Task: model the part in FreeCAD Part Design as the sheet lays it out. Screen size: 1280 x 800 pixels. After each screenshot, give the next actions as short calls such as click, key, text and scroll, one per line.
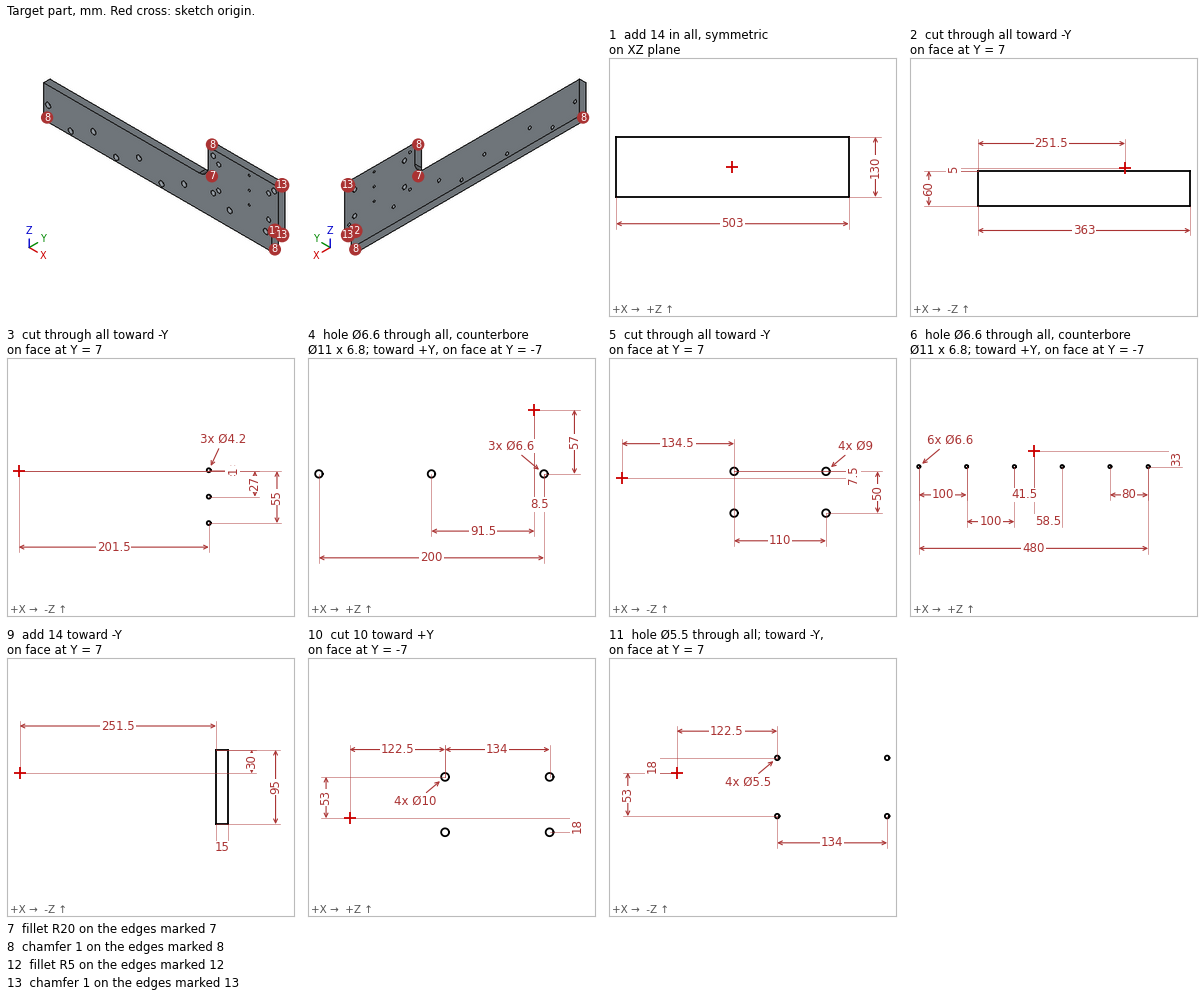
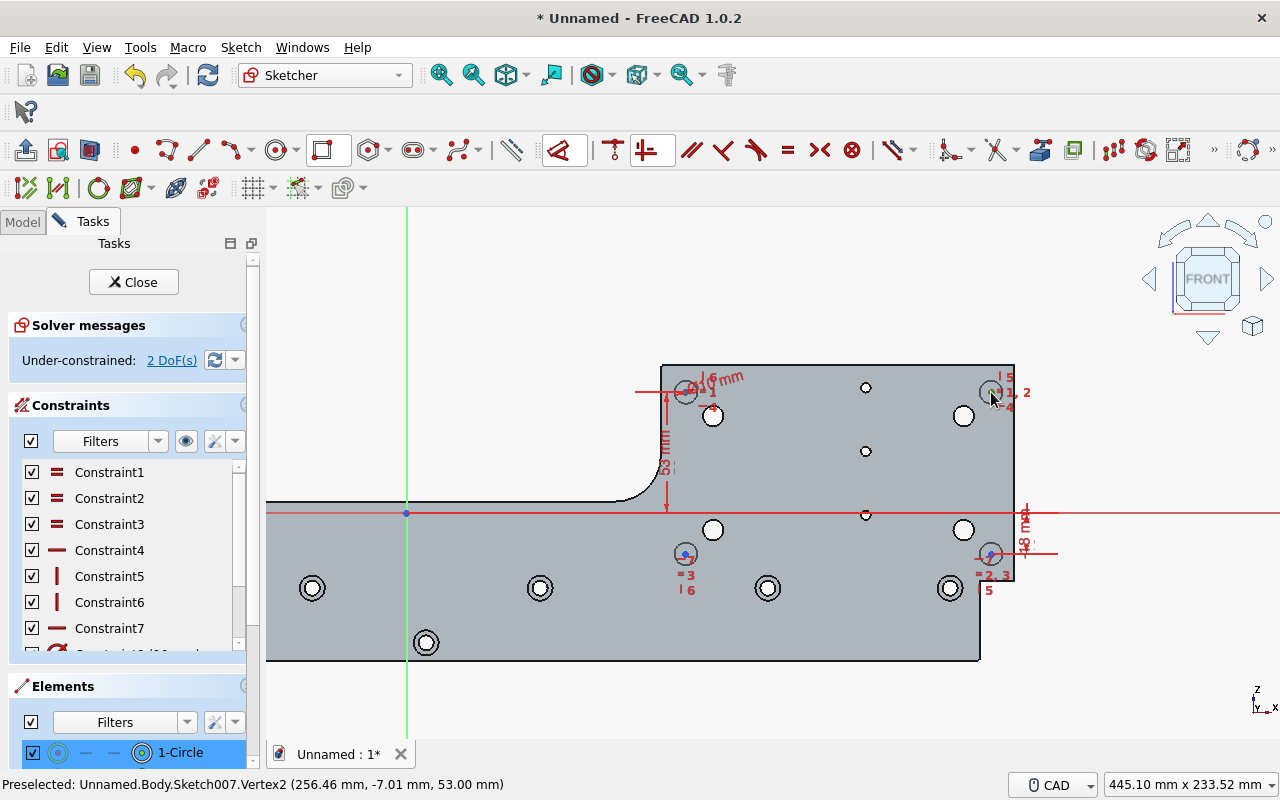
key(l)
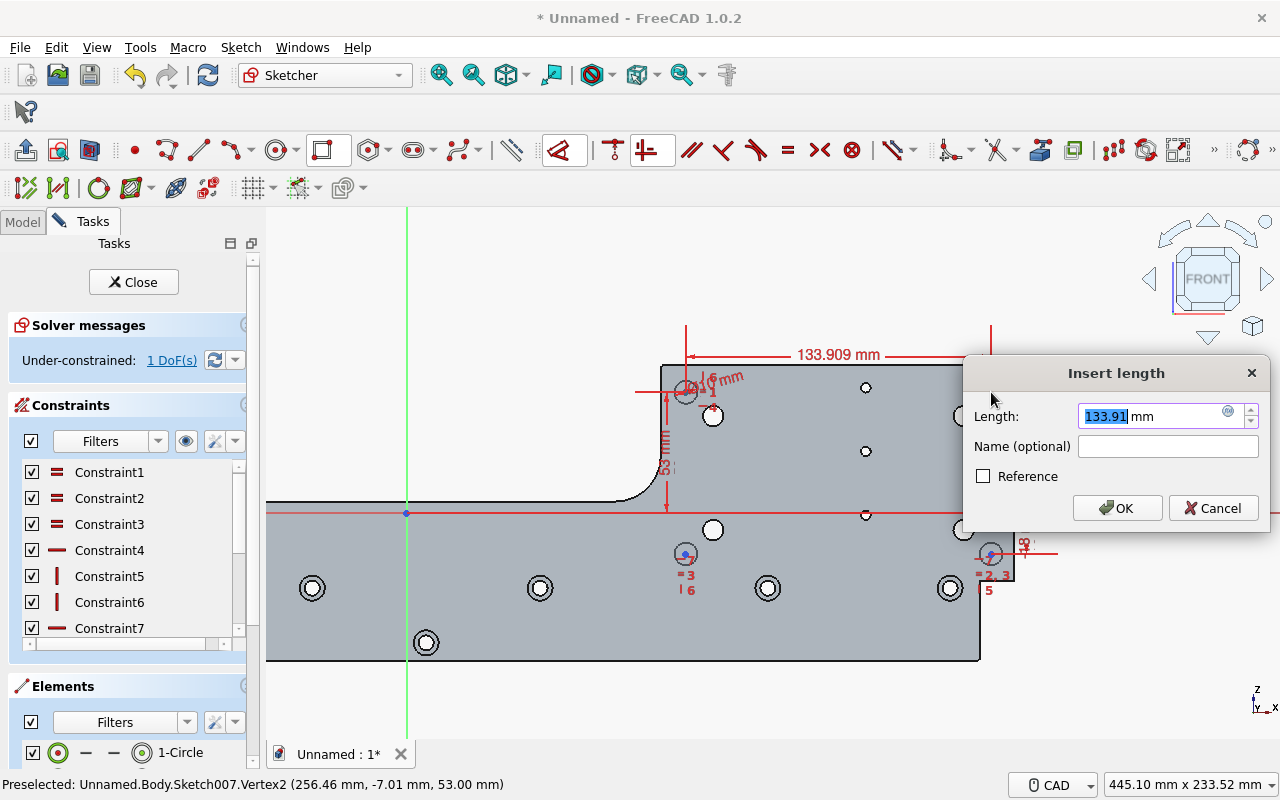
text(134)
key(Return)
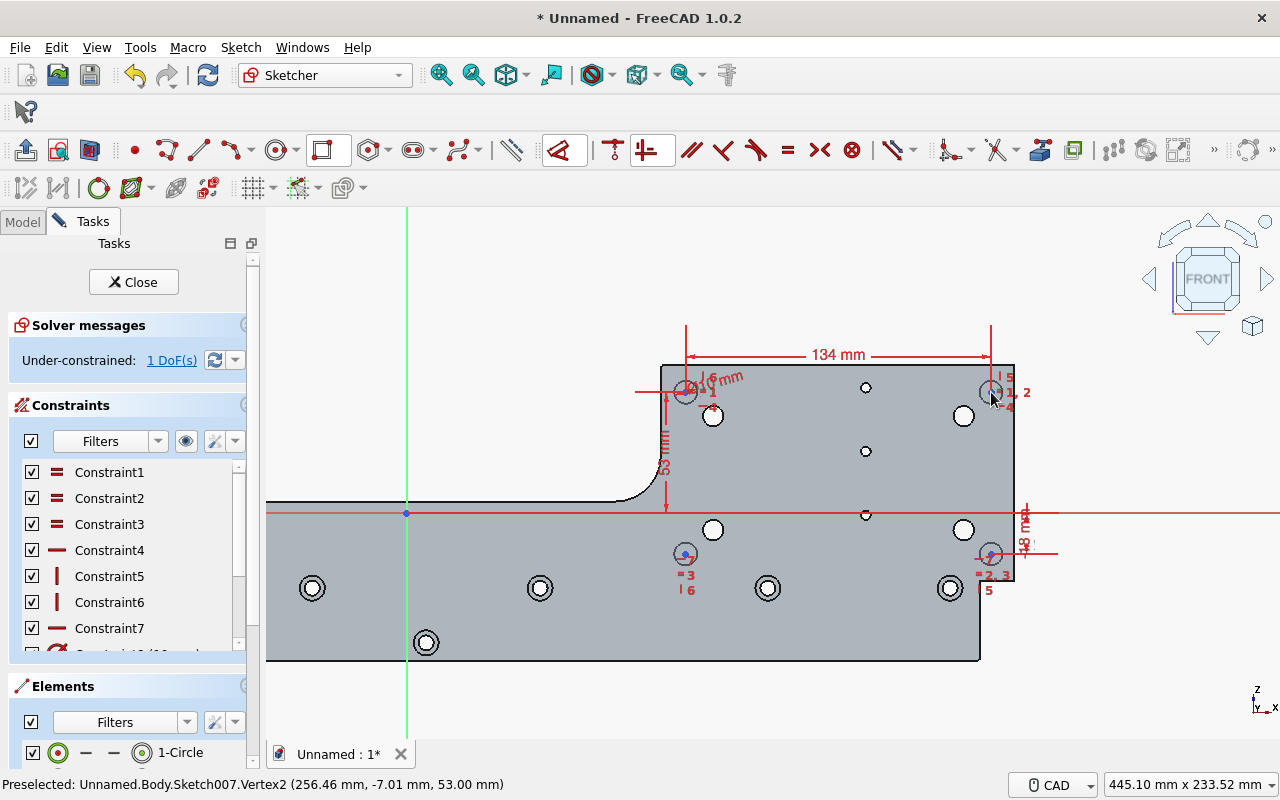
click(686, 392)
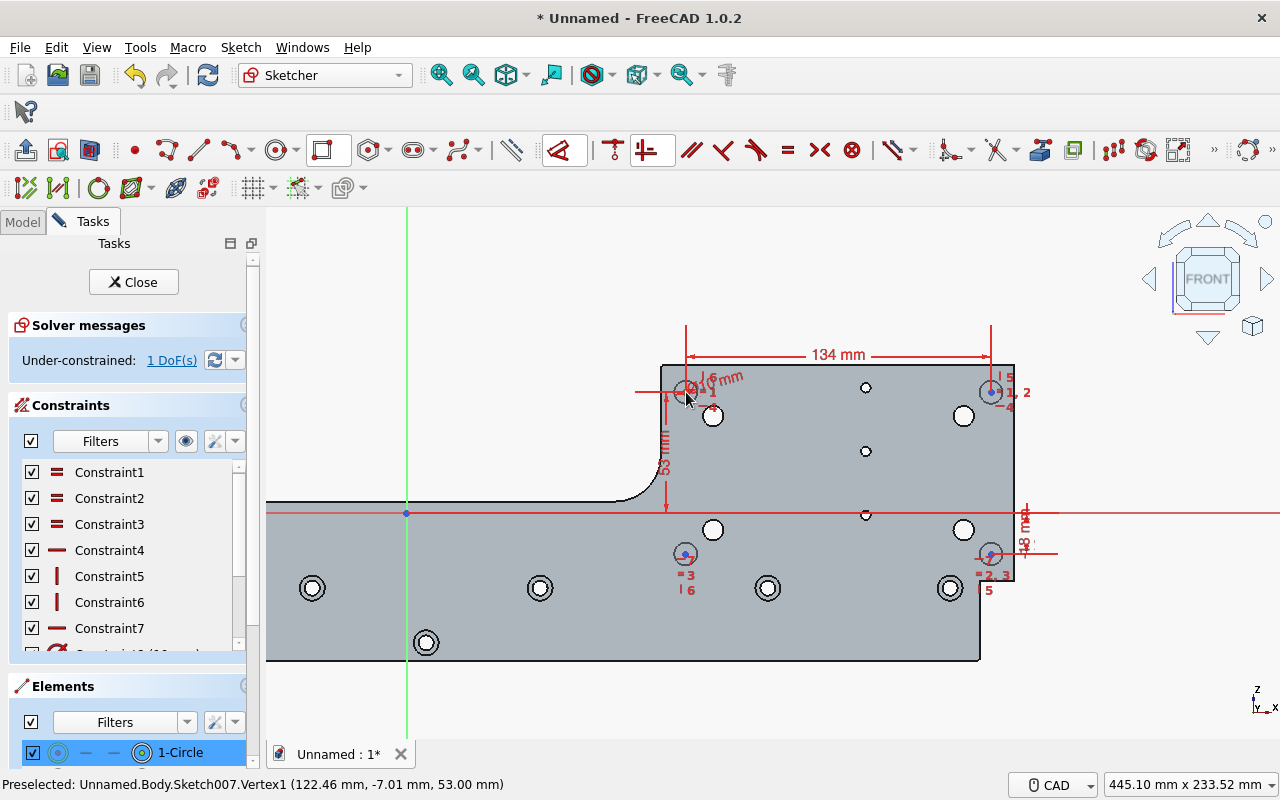
key(l)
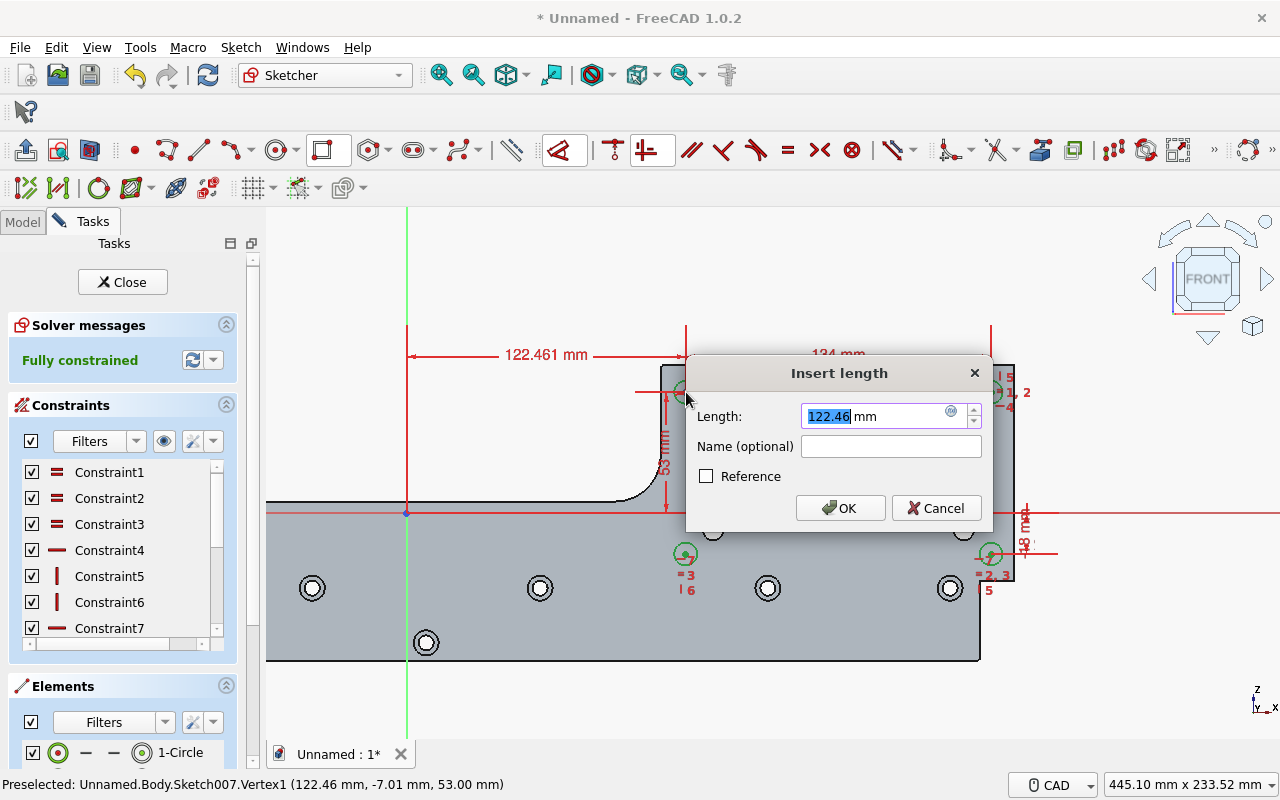
text(122.5)
key(Return)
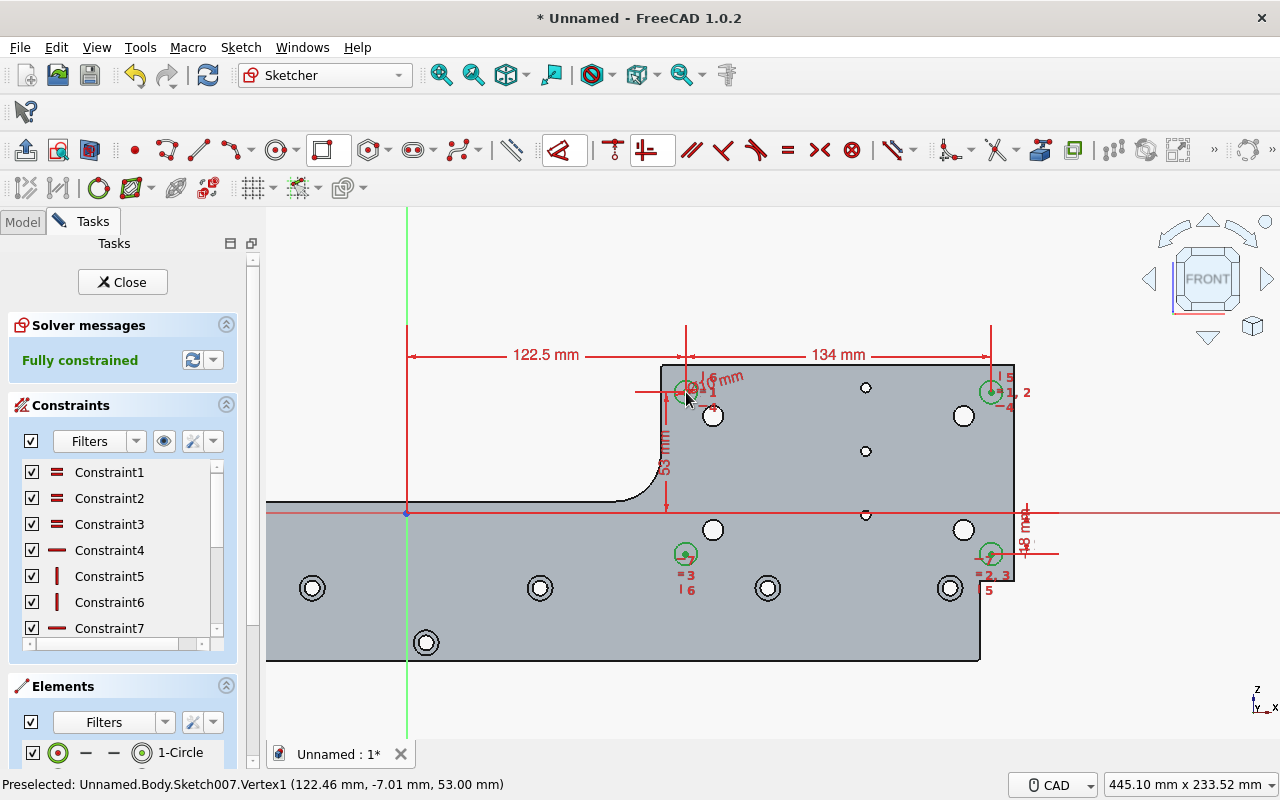
click(123, 282)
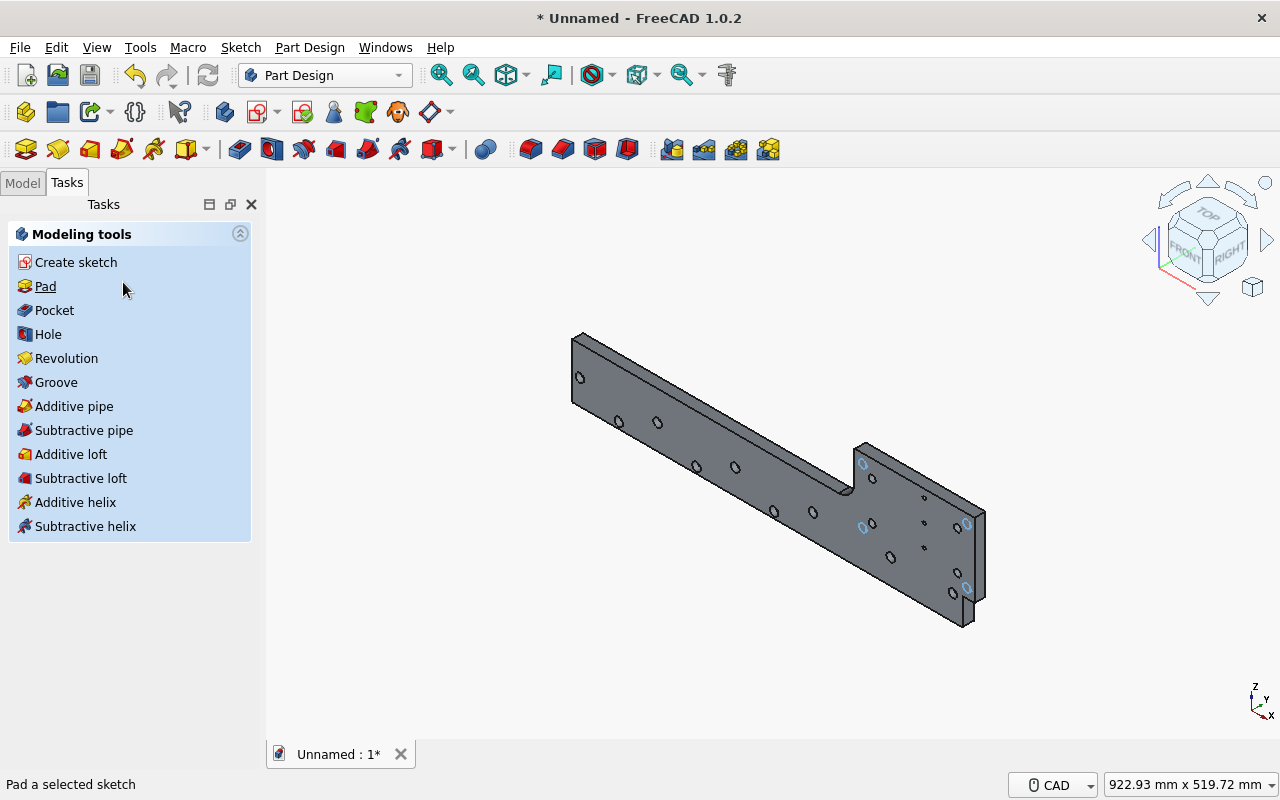
click(240, 150)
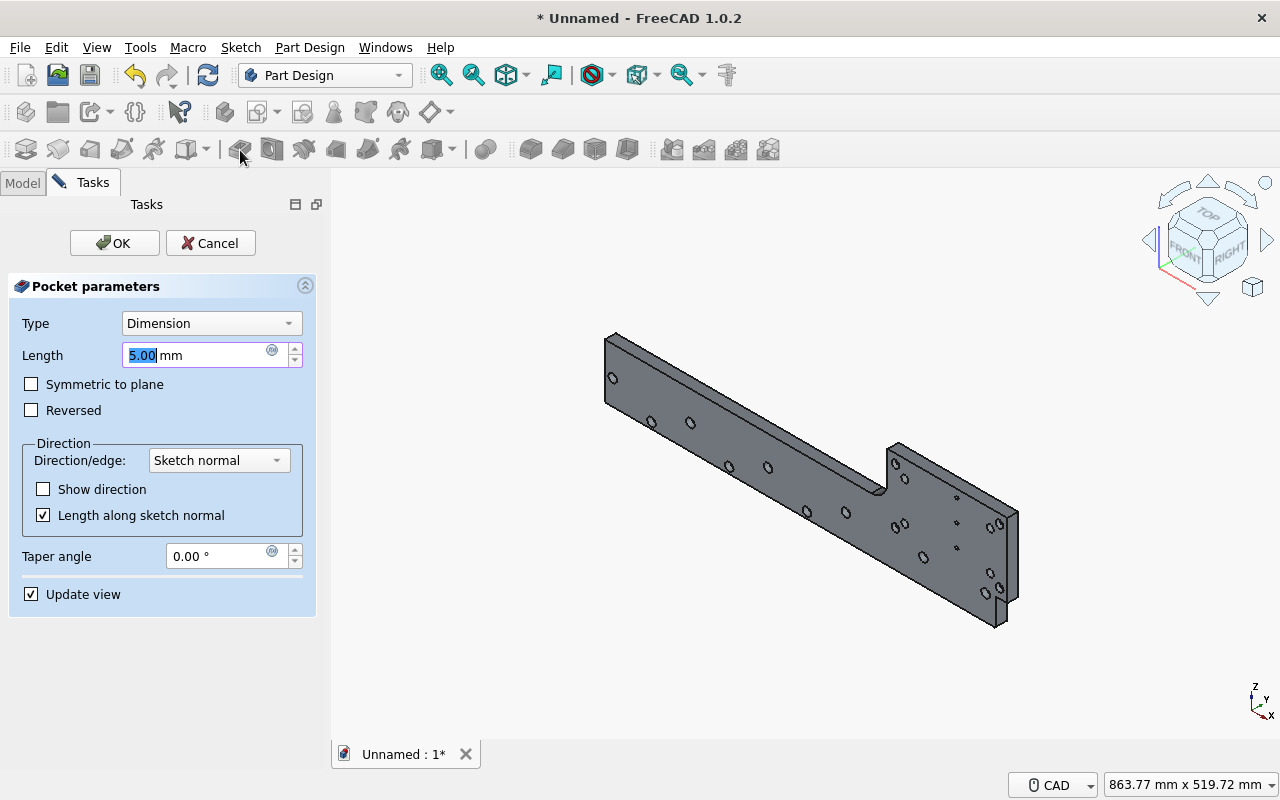
text(10)
key(Tab)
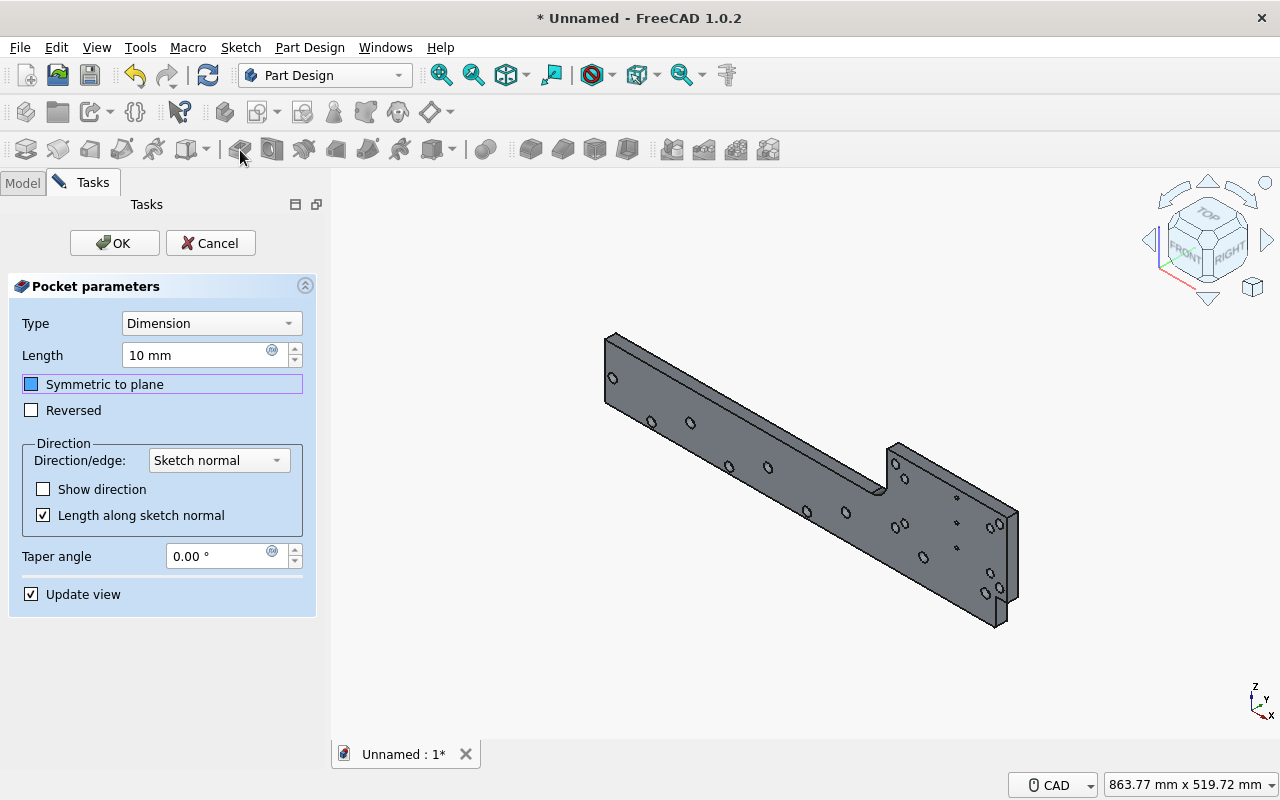
click(115, 243)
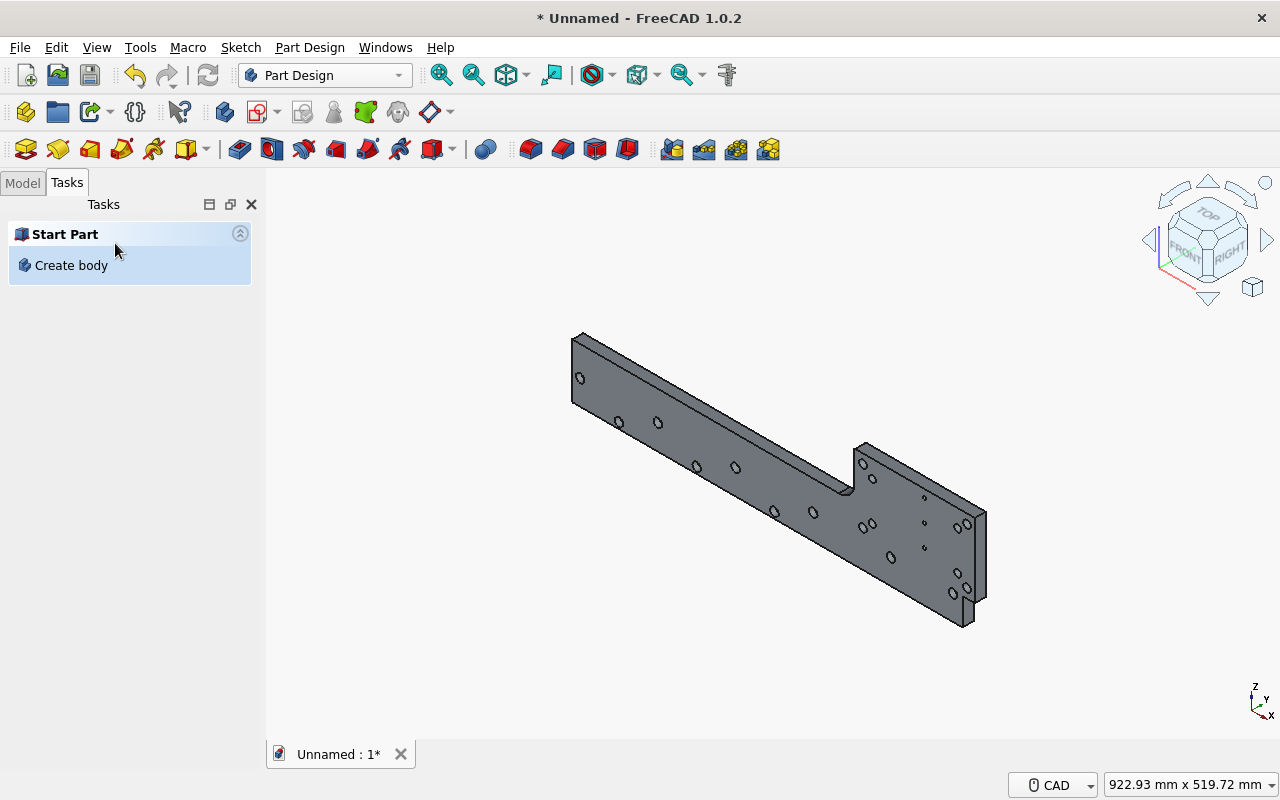
key(4)